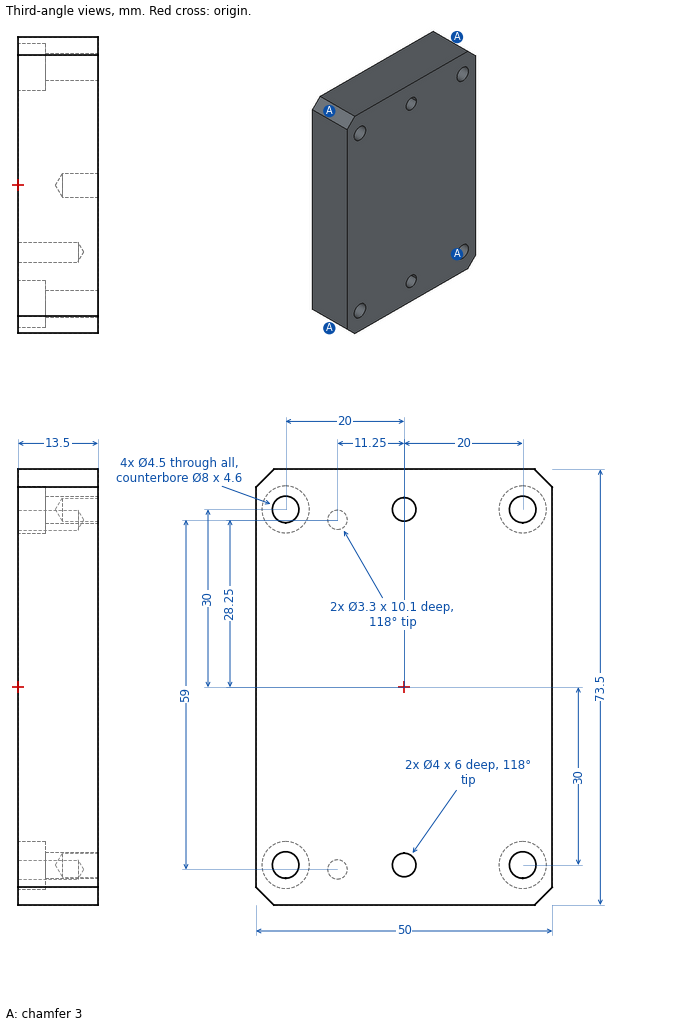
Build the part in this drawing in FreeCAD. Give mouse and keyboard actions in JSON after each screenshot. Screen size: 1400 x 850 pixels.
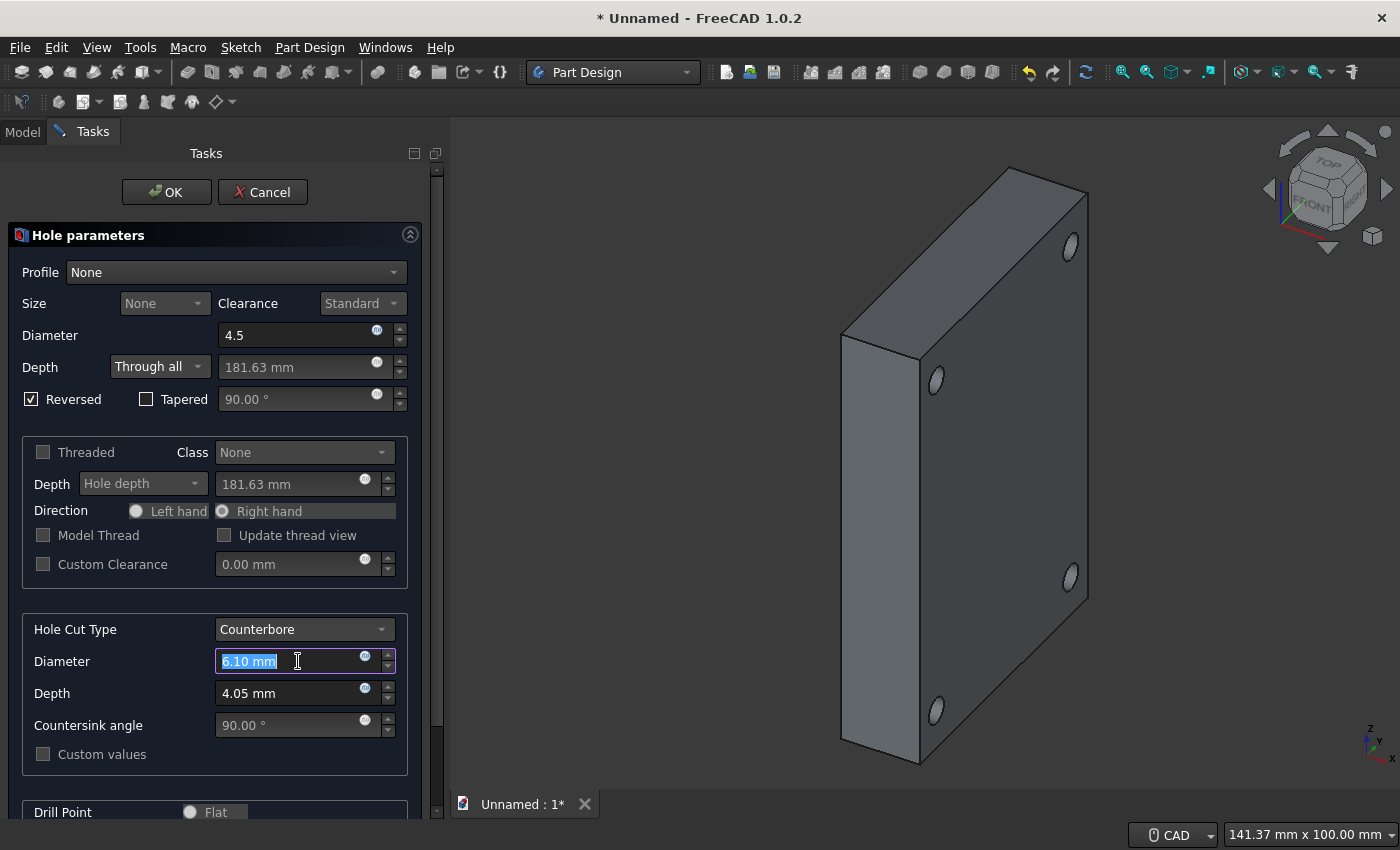
{"action": "type", "text": "8"}
{"action": "key", "text": "Tab"}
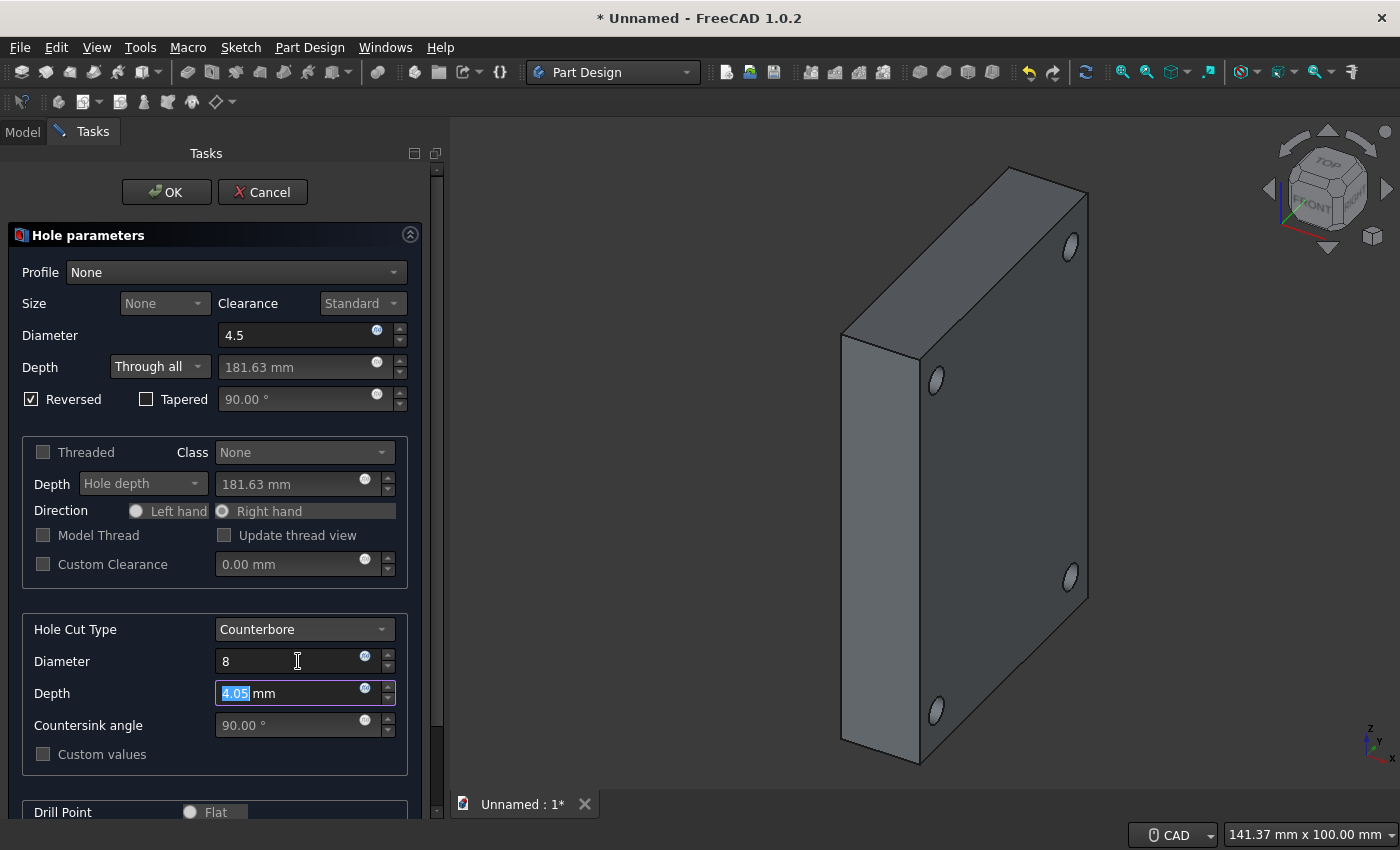
{"action": "type", "text": "4.6"}
{"action": "key", "text": "Tab"}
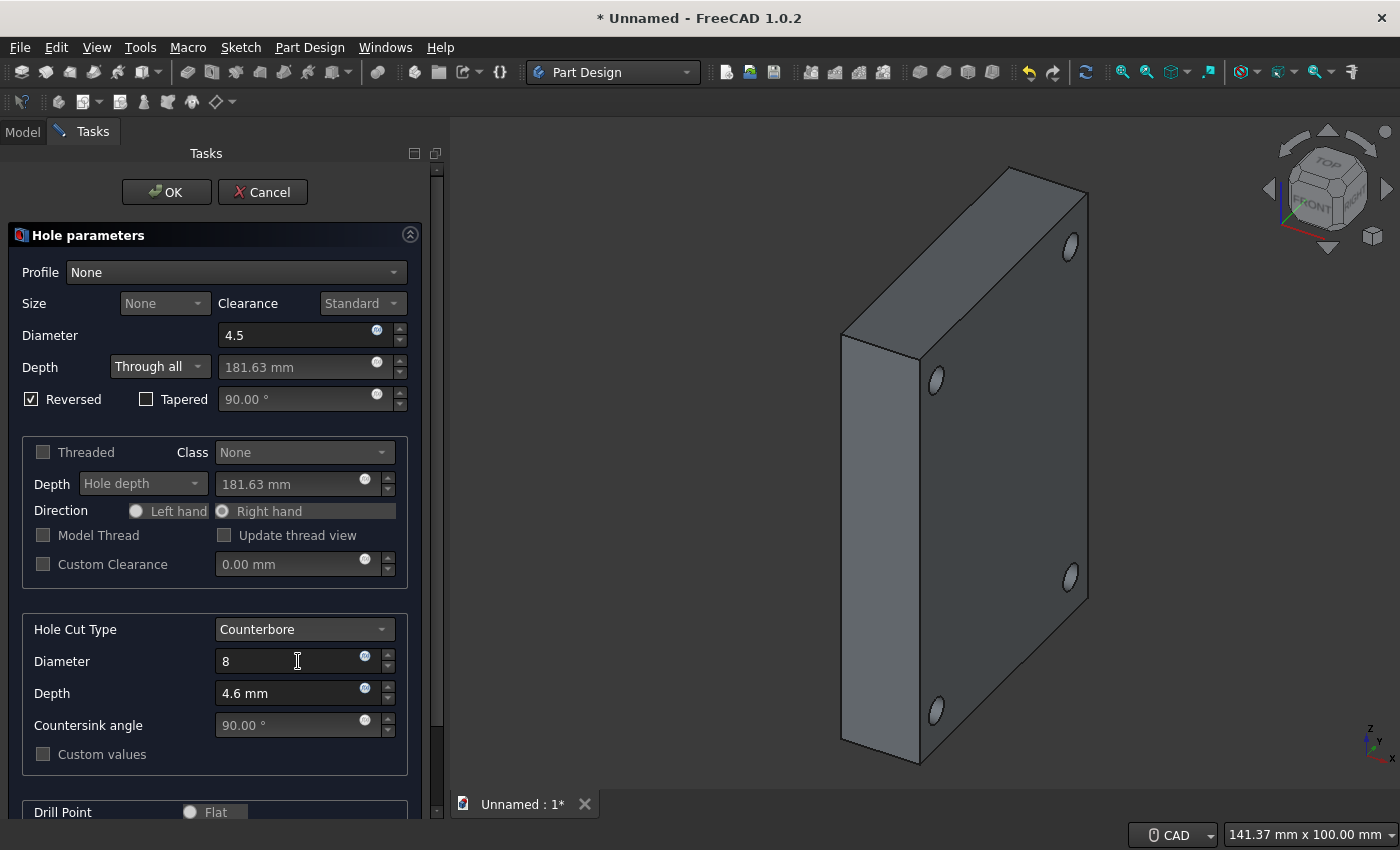
{"action": "left_click", "coordinate": [167, 192]}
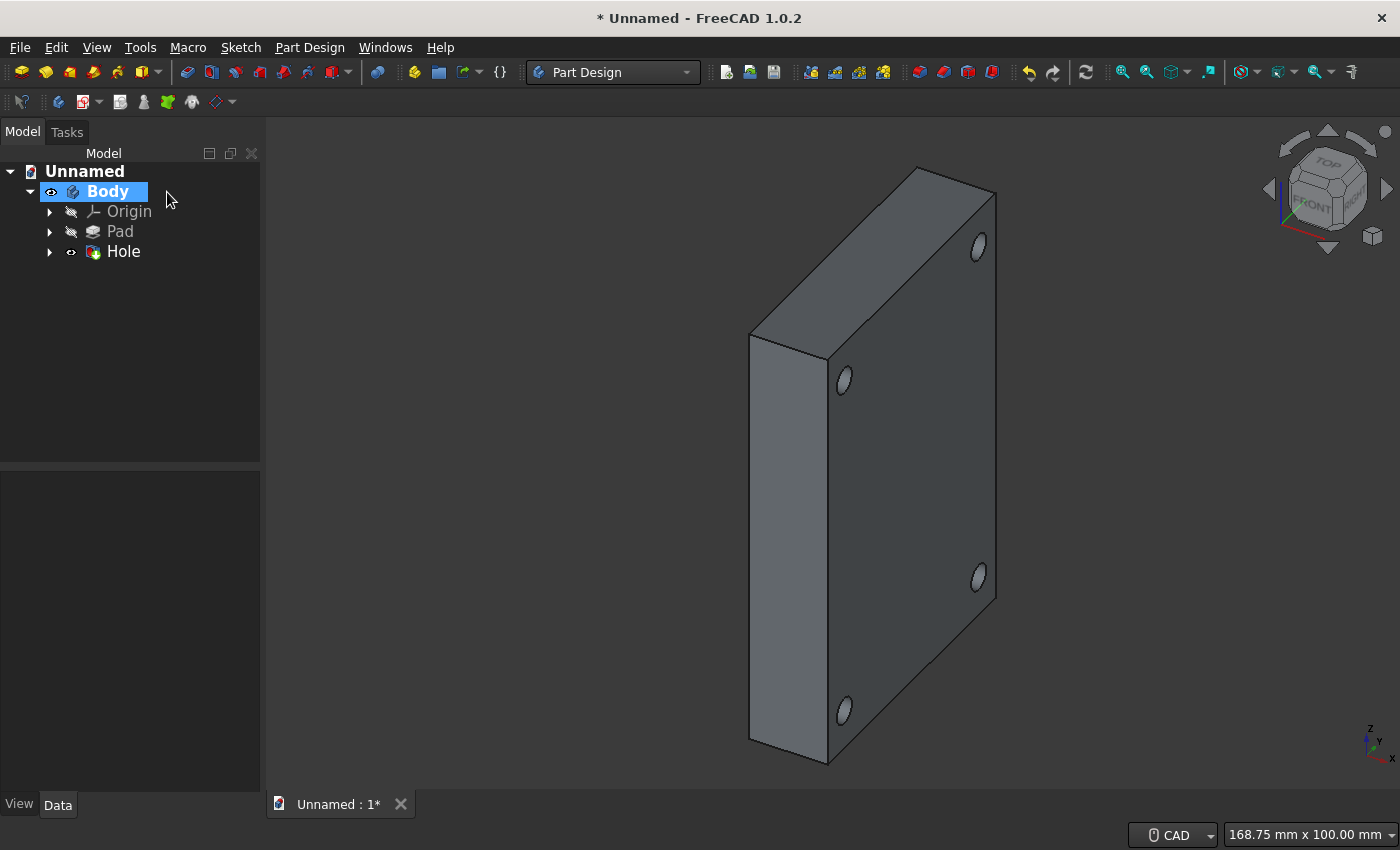
{"action": "left_click", "coordinate": [912, 536]}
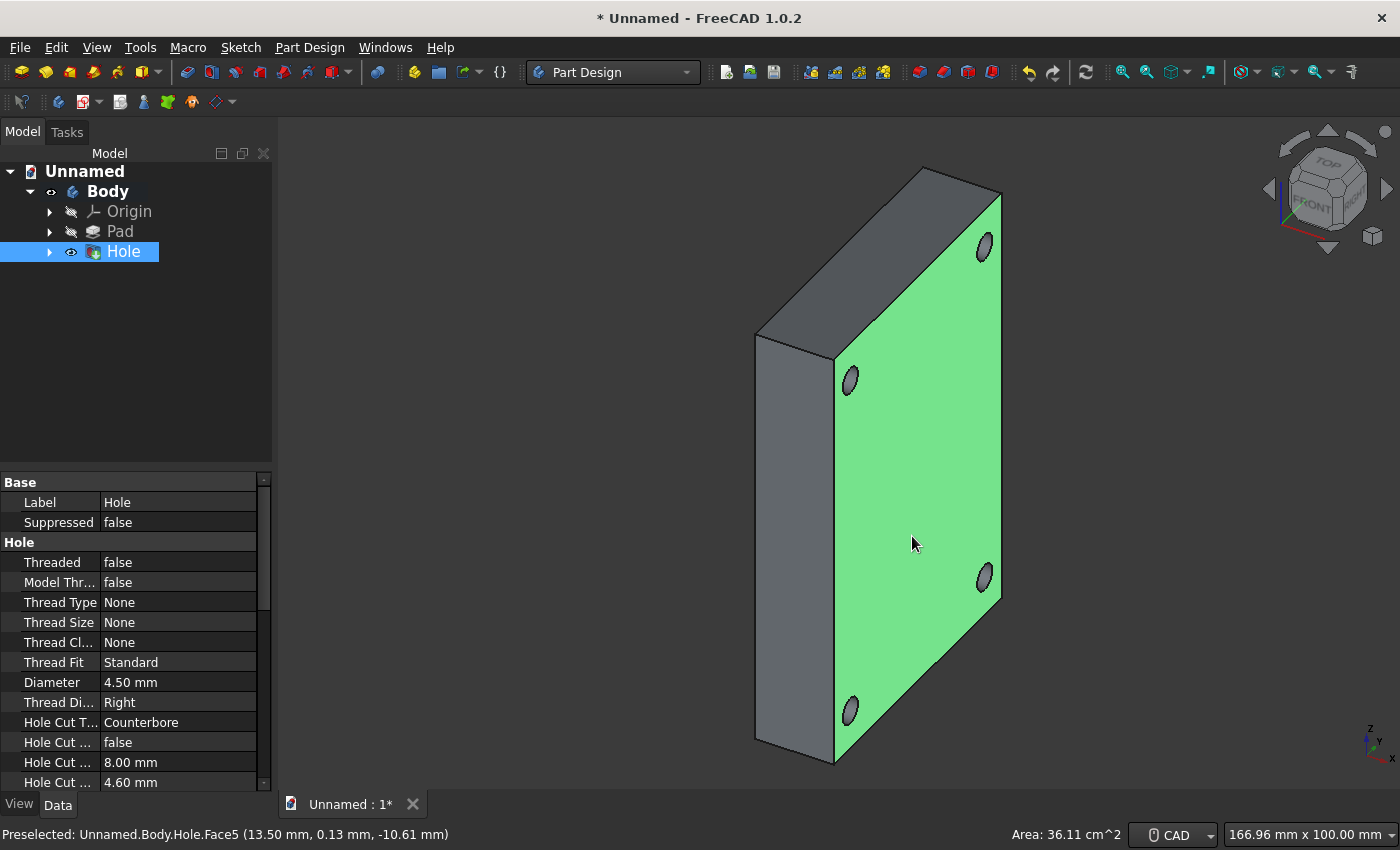
{"action": "left_click", "coordinate": [84, 102]}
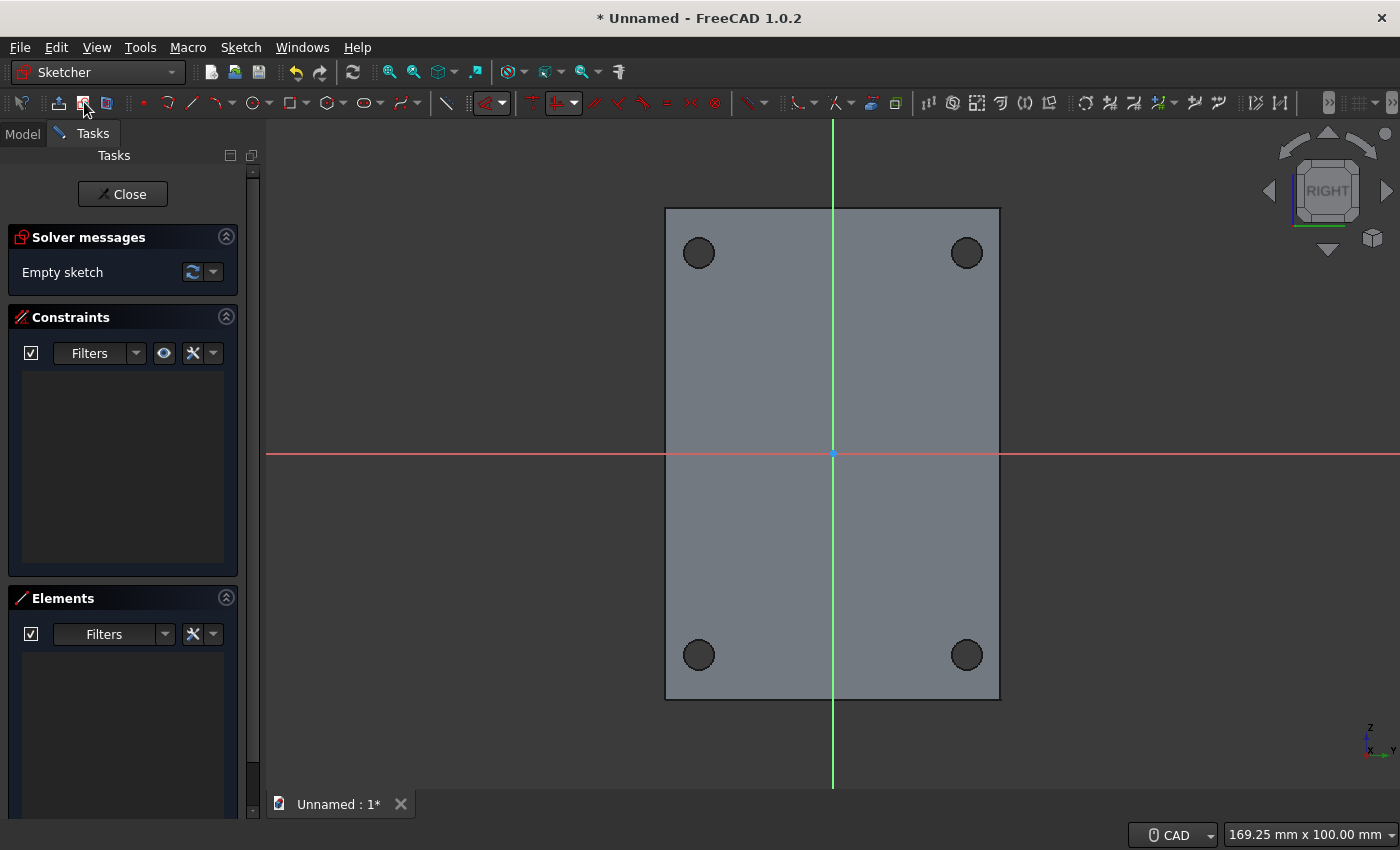
{"action": "left_click", "coordinate": [254, 104]}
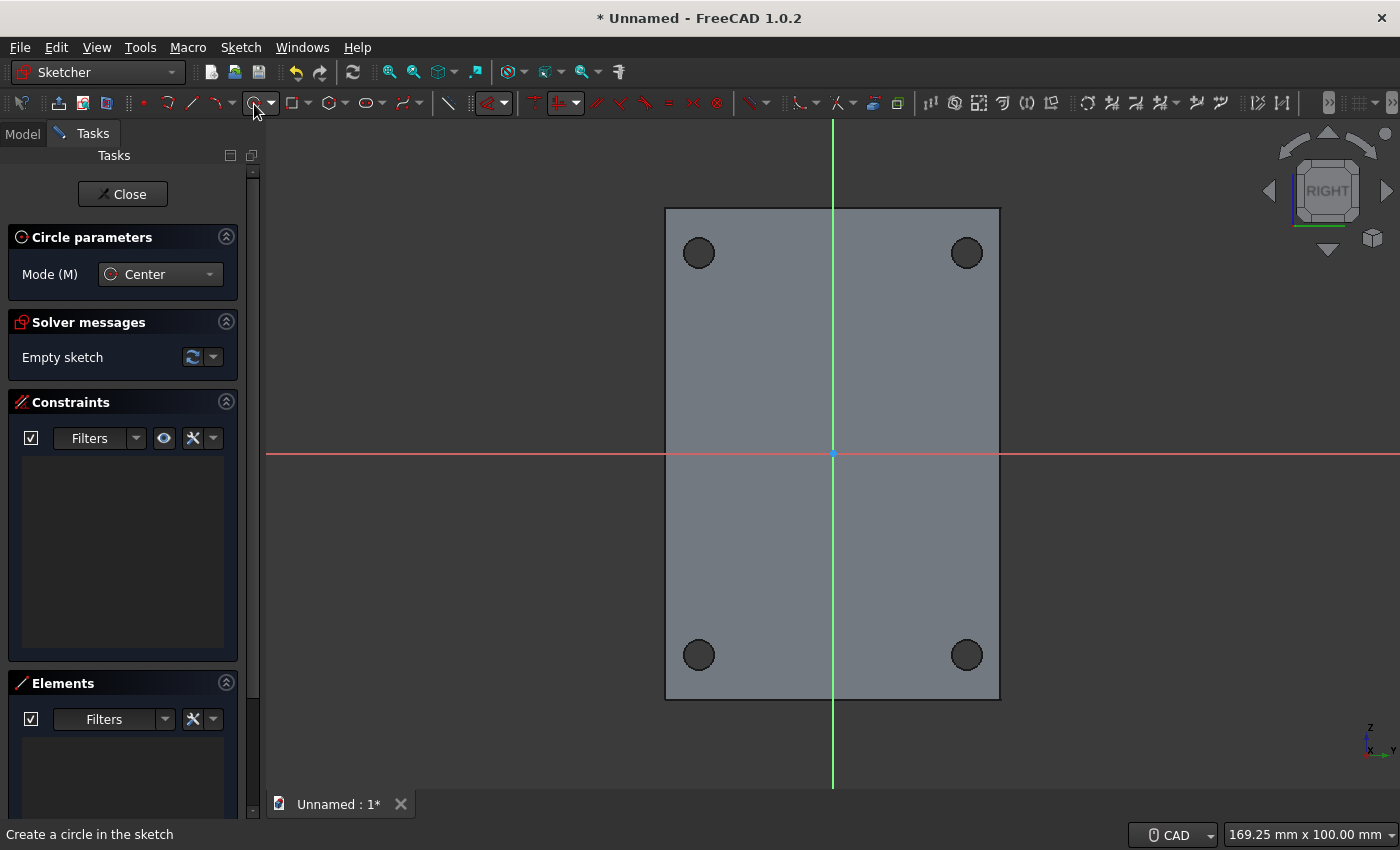
{"action": "scroll", "coordinate": [833, 655], "scroll_direction": "up", "scroll_amount": 3}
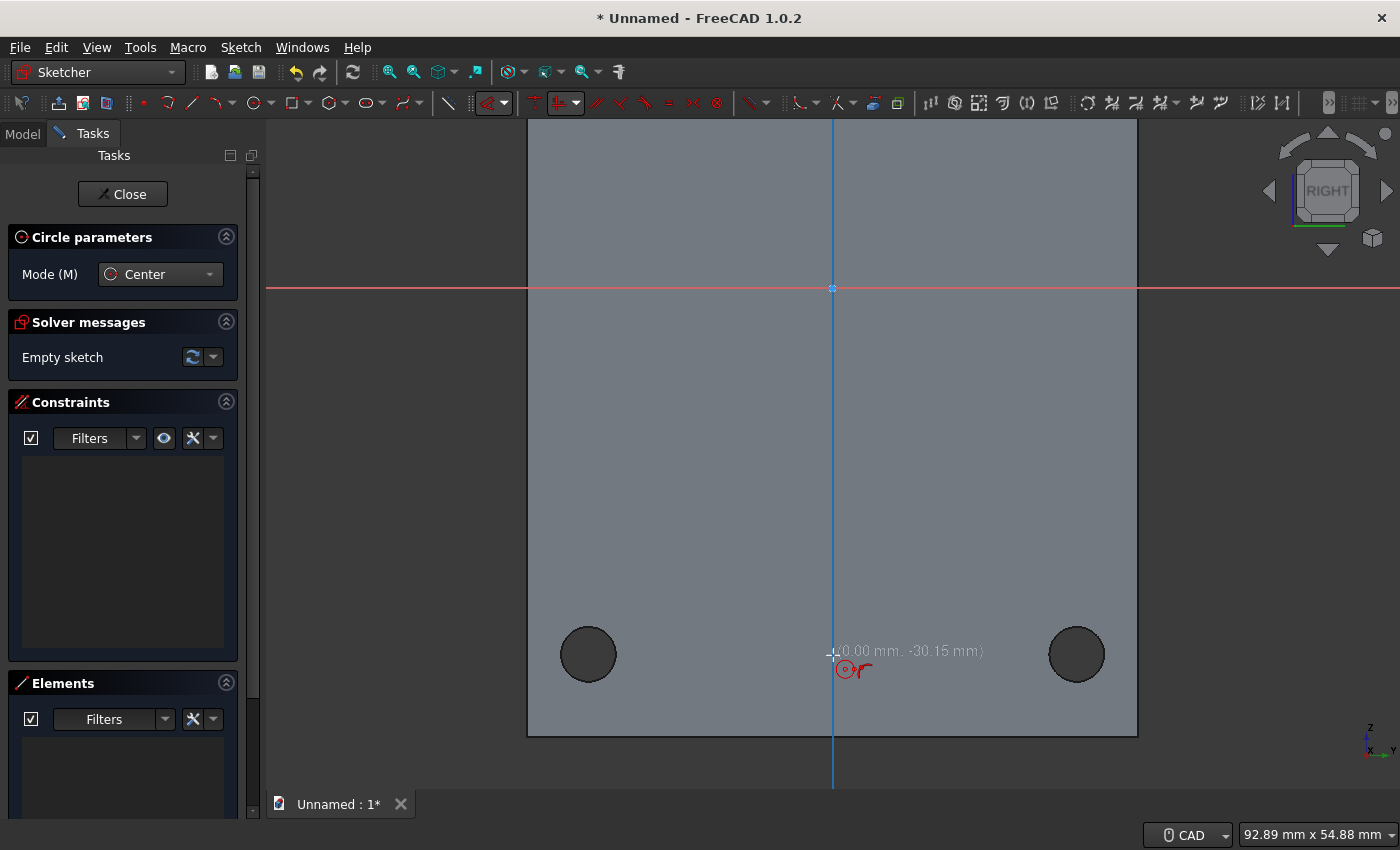
{"action": "left_click", "coordinate": [833, 654]}
{"action": "mouse_move", "coordinate": [850, 637]}